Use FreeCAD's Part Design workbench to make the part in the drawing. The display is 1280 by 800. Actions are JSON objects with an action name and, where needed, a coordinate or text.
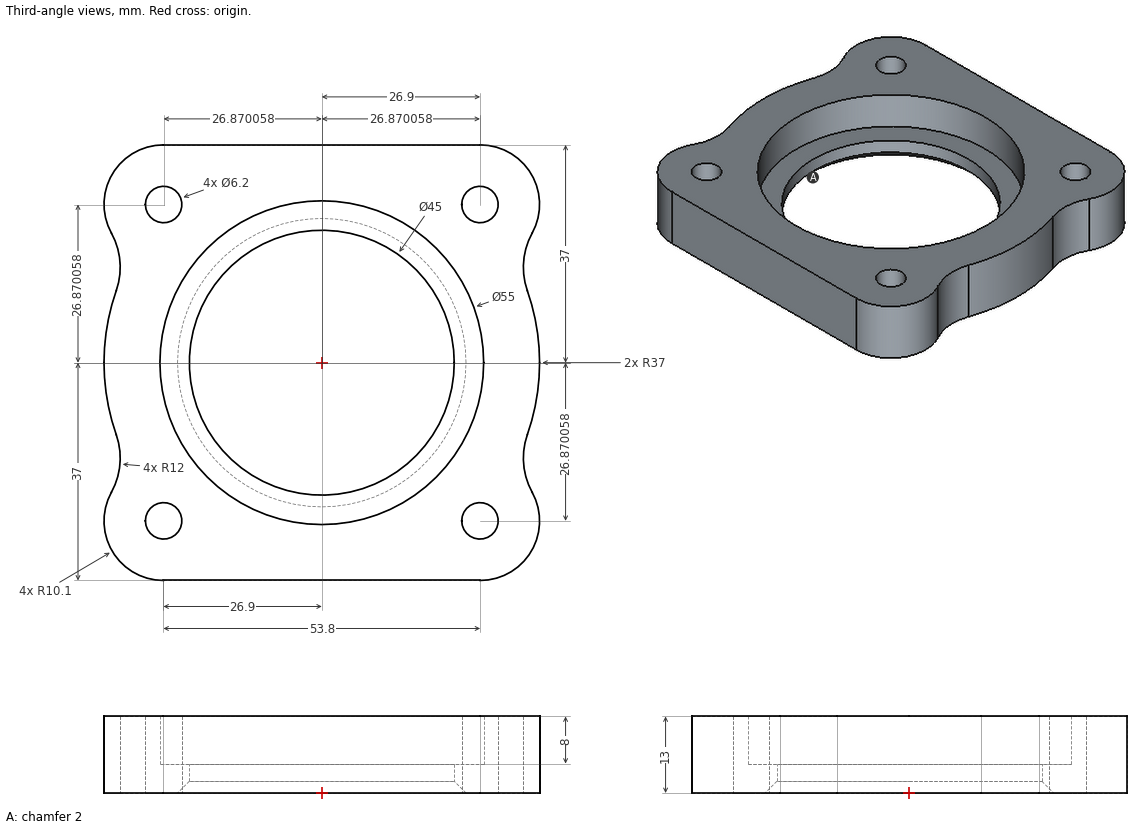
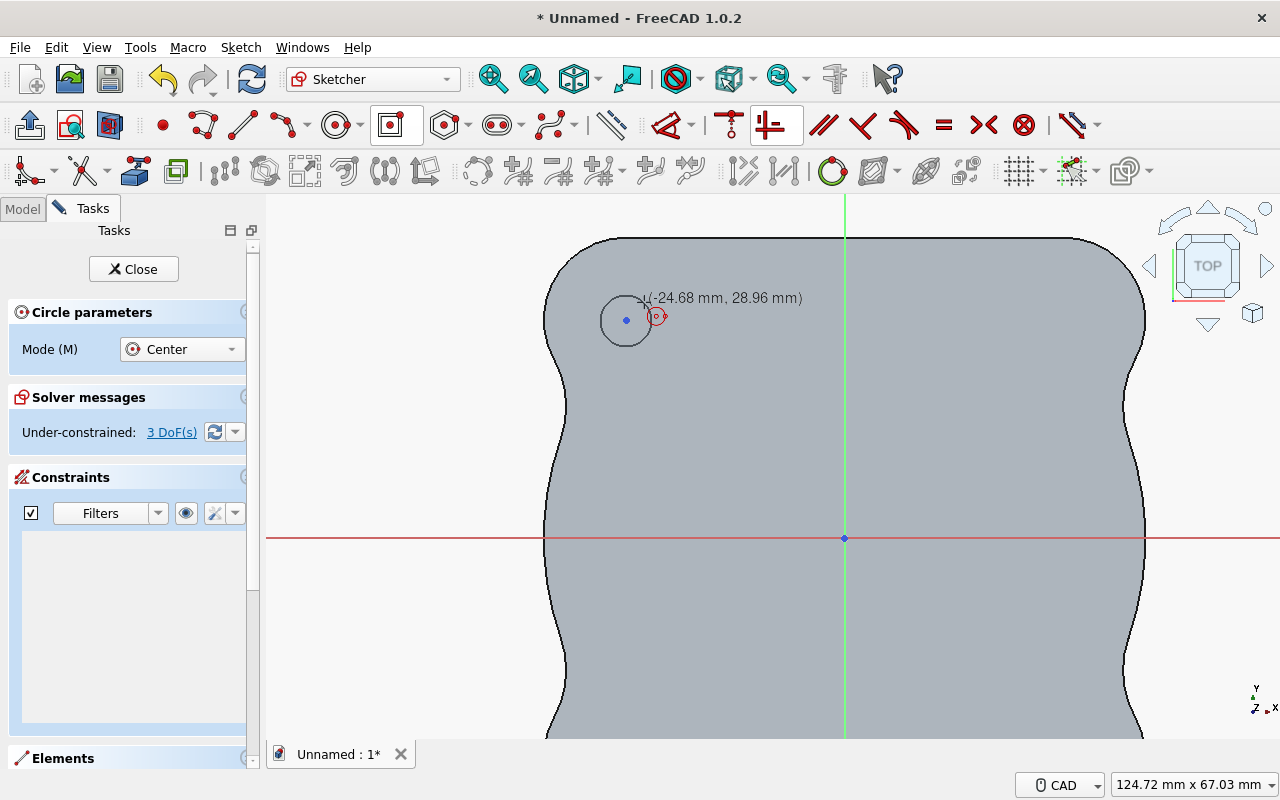
{"action": "left_click", "coordinate": [1063, 320]}
{"action": "left_click", "coordinate": [1081, 302]}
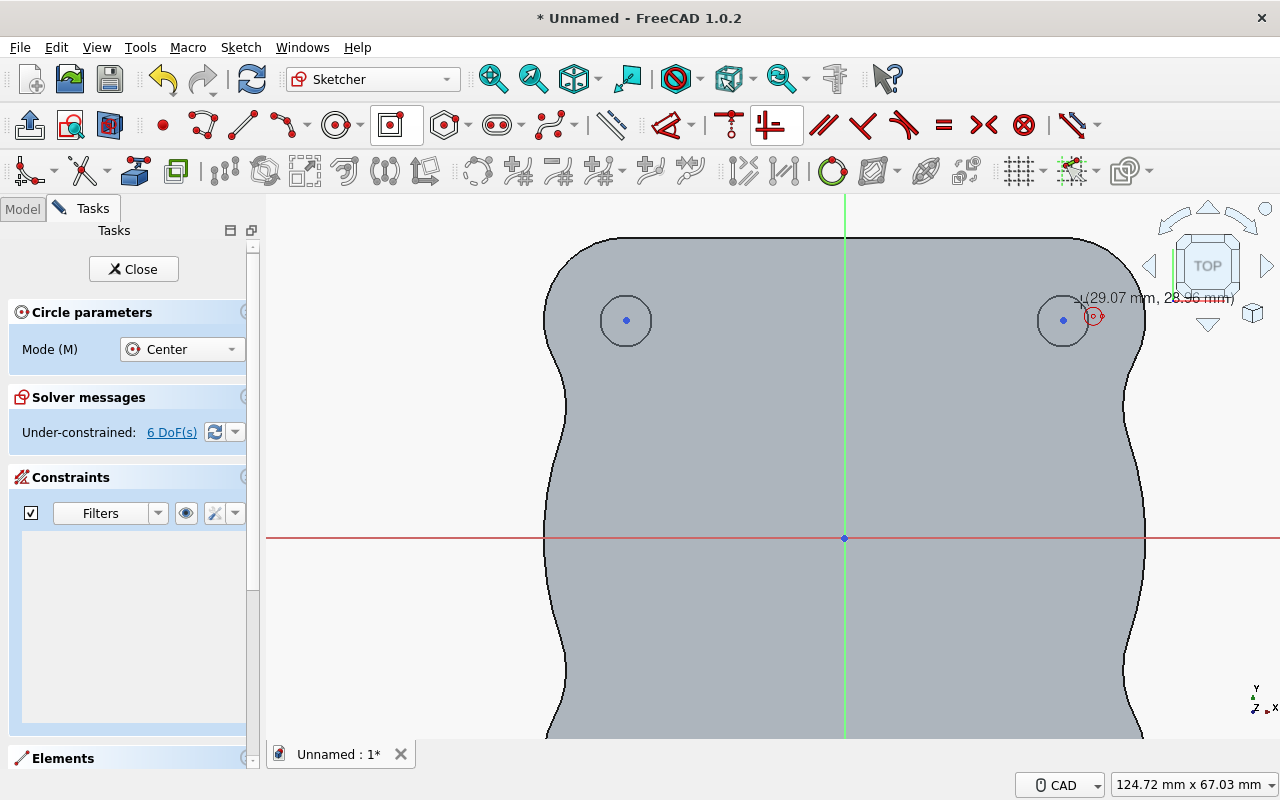
{"action": "scroll", "coordinate": [420, 320], "scroll_direction": "down", "scroll_amount": 2}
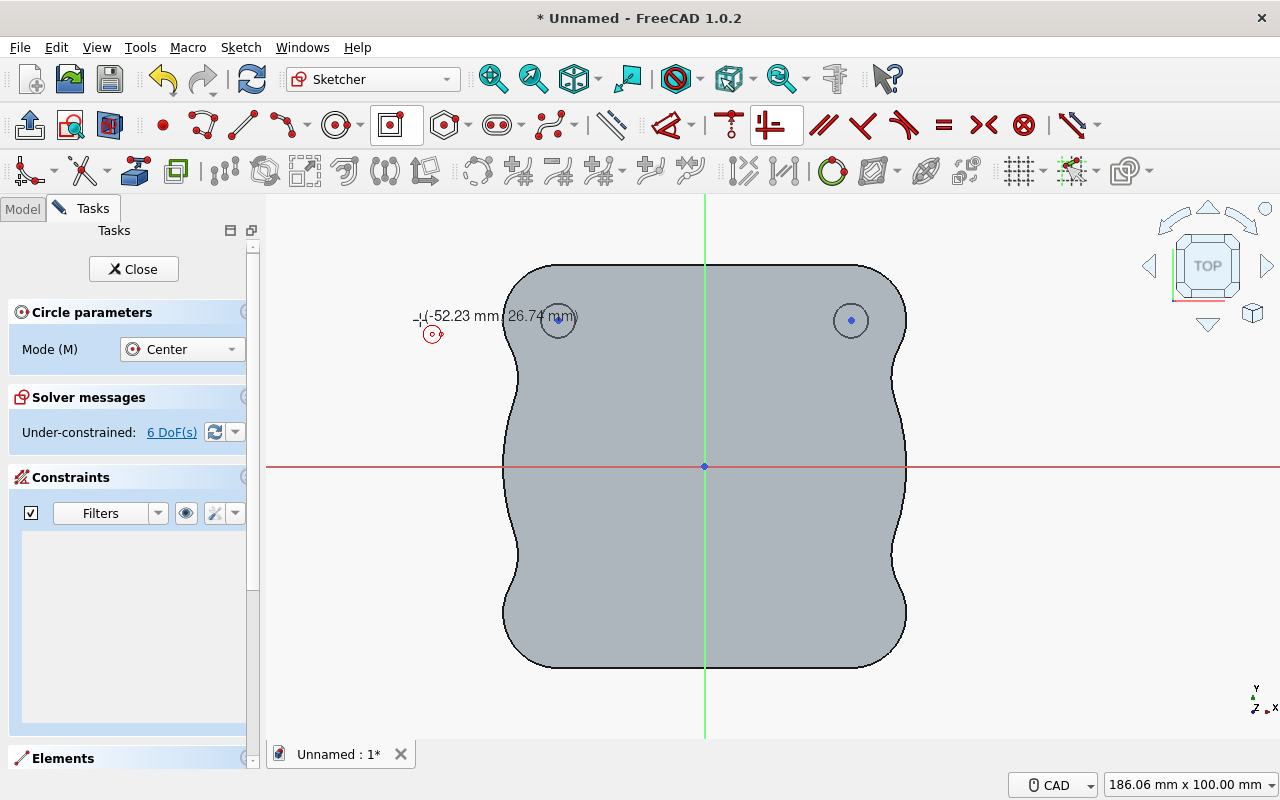
{"action": "scroll", "coordinate": [851, 613], "scroll_direction": "up", "scroll_amount": 2}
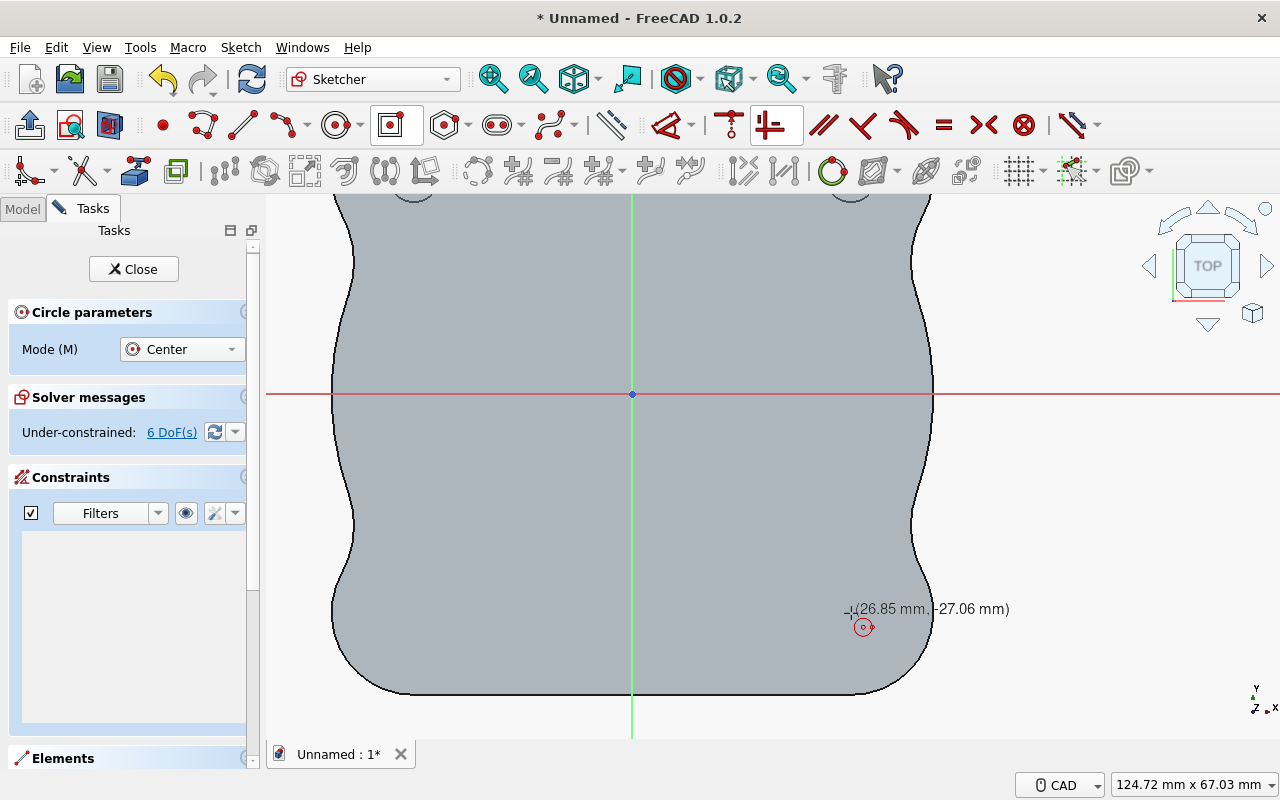
{"action": "left_click", "coordinate": [851, 613]}
{"action": "left_click", "coordinate": [869, 595]}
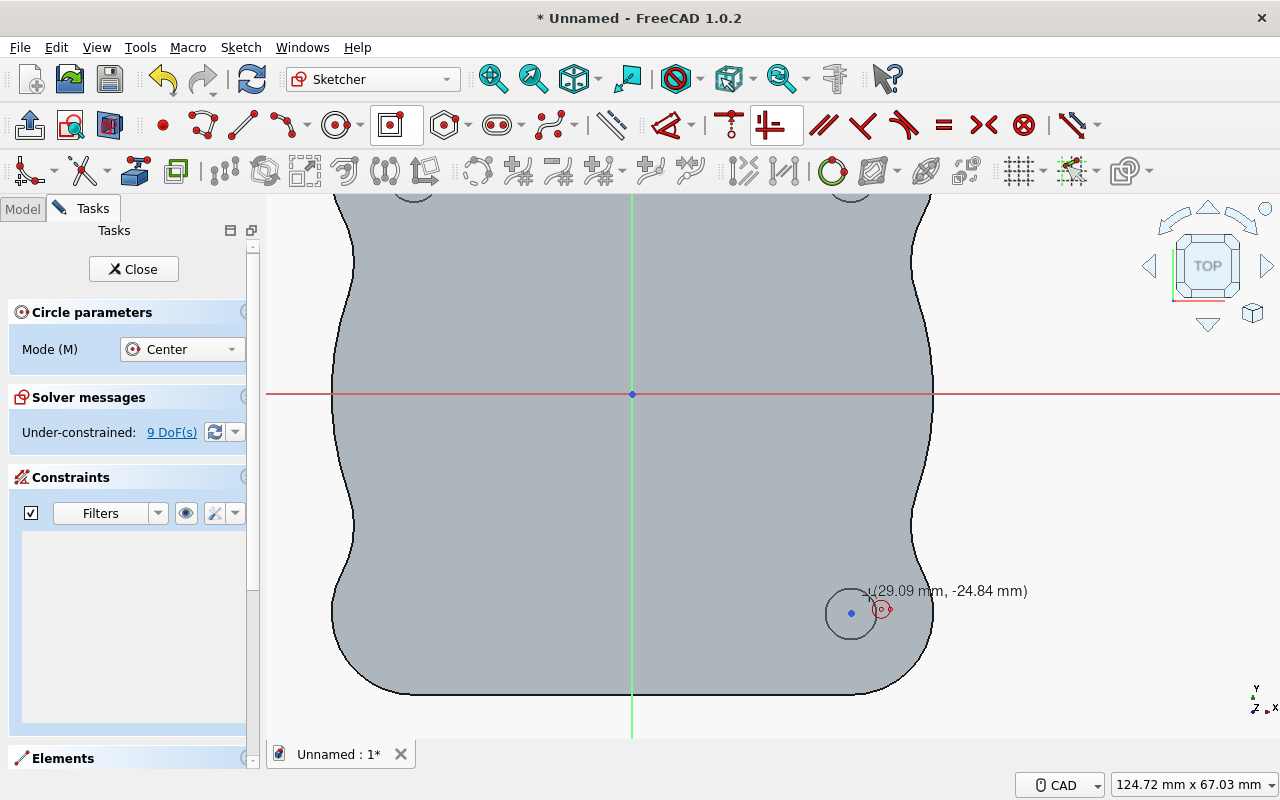
{"action": "left_click", "coordinate": [414, 613]}
{"action": "left_click", "coordinate": [432, 595]}
{"action": "key", "text": "Escape"}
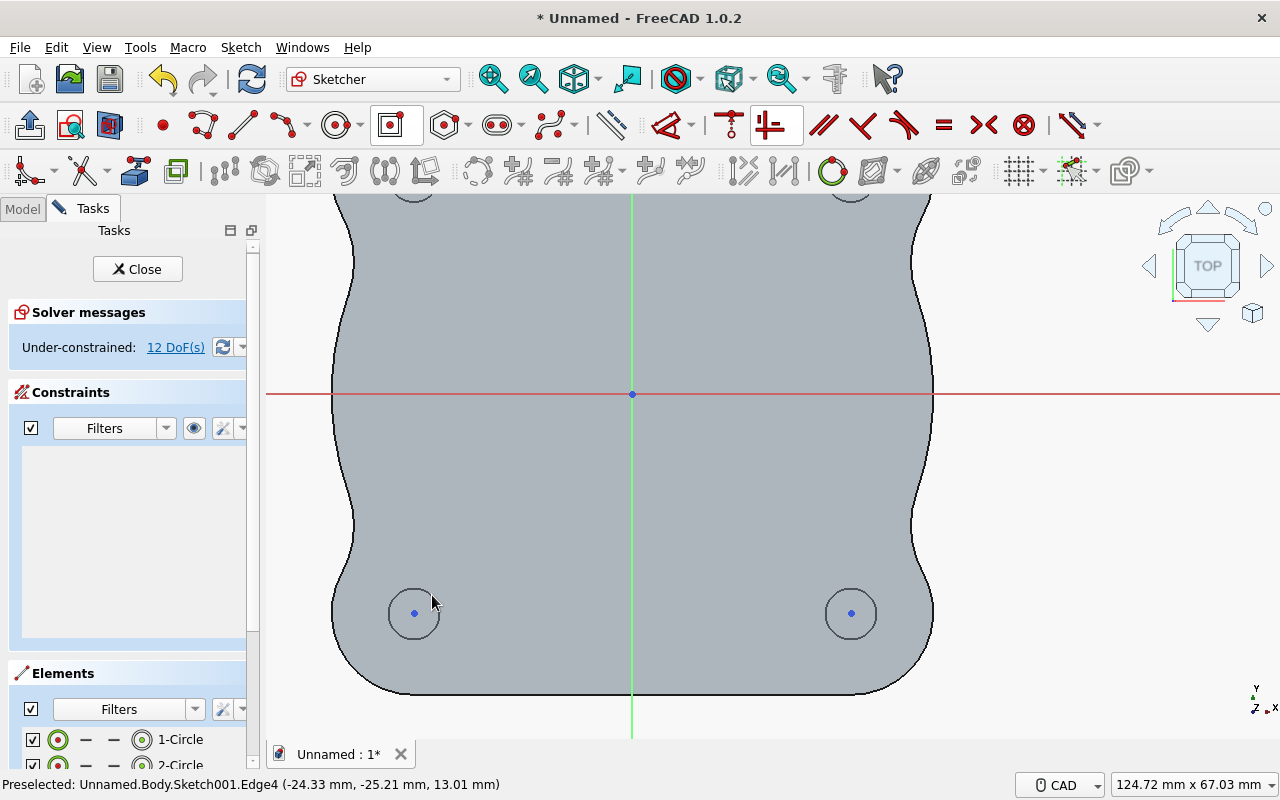
{"action": "scroll", "coordinate": [851, 614], "scroll_direction": "down", "scroll_amount": 2}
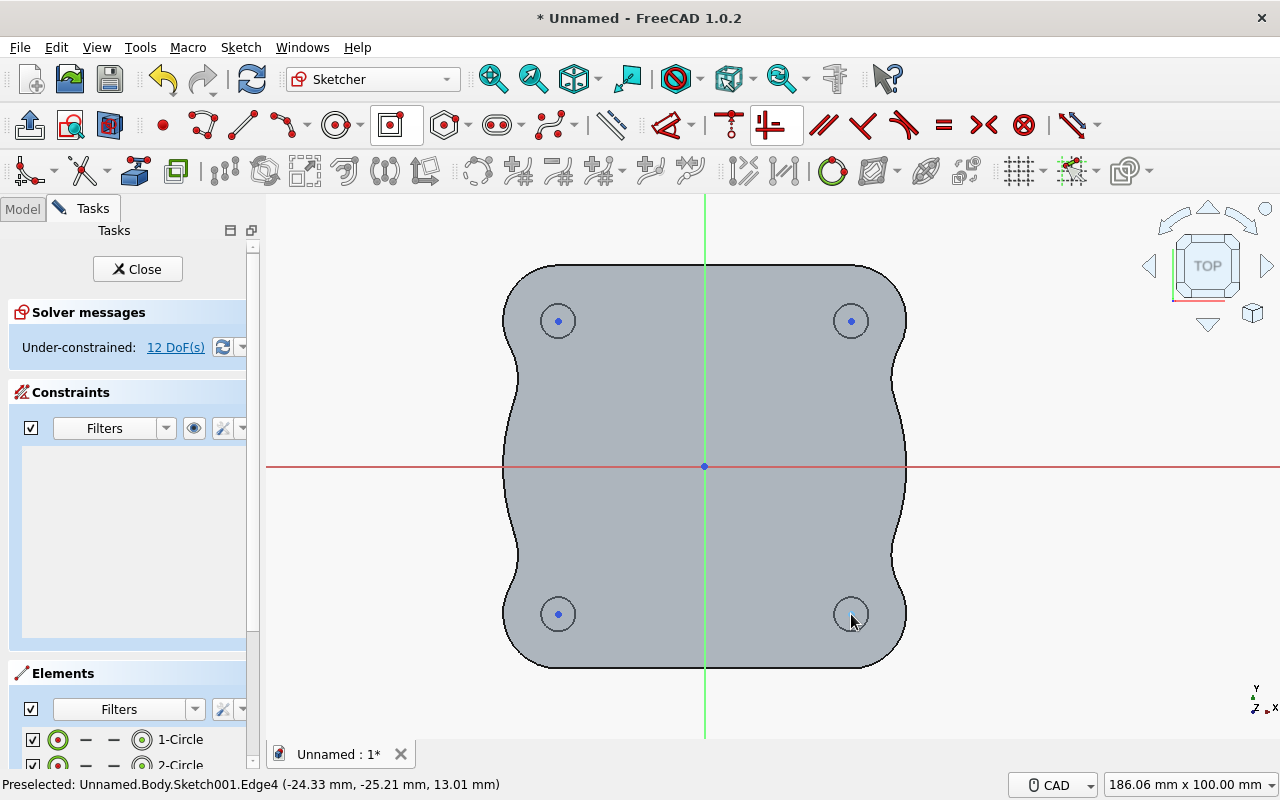
{"action": "left_click", "coordinate": [570, 309]}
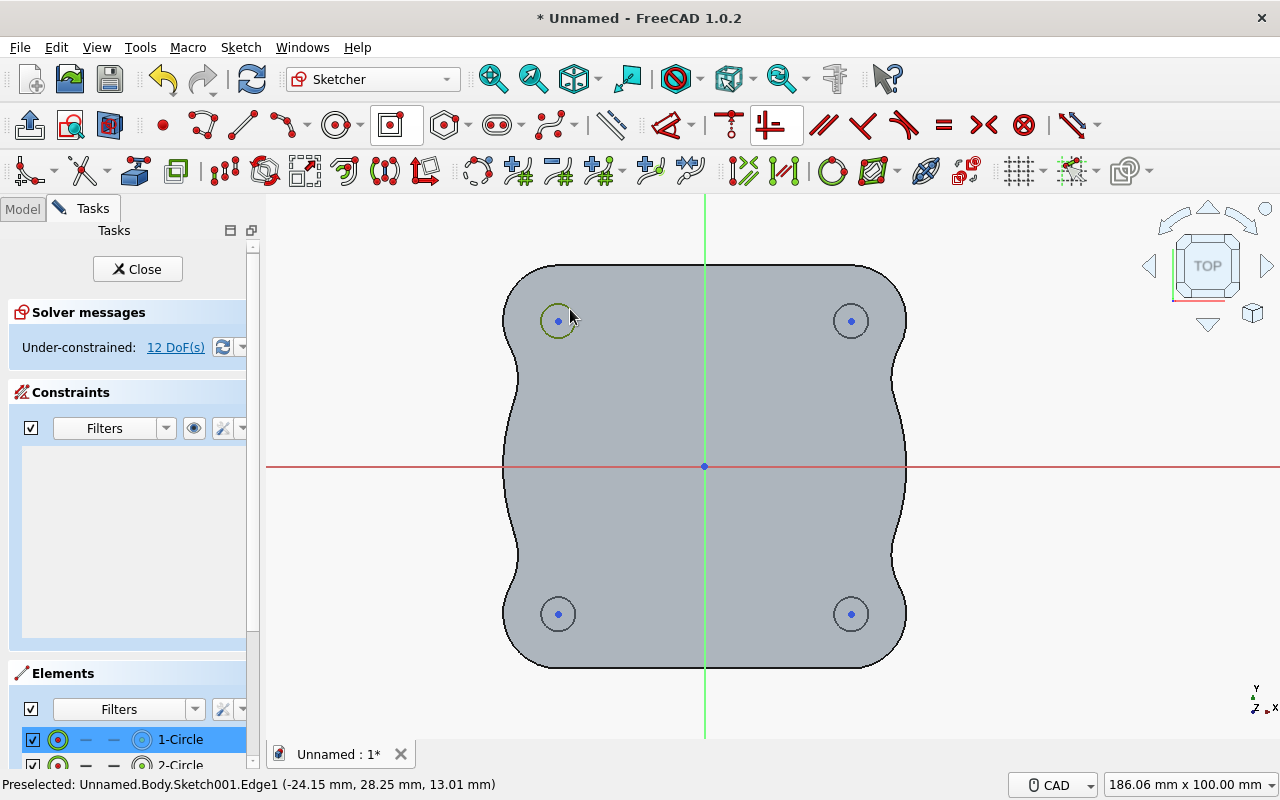
{"action": "left_click", "coordinate": [863, 309]}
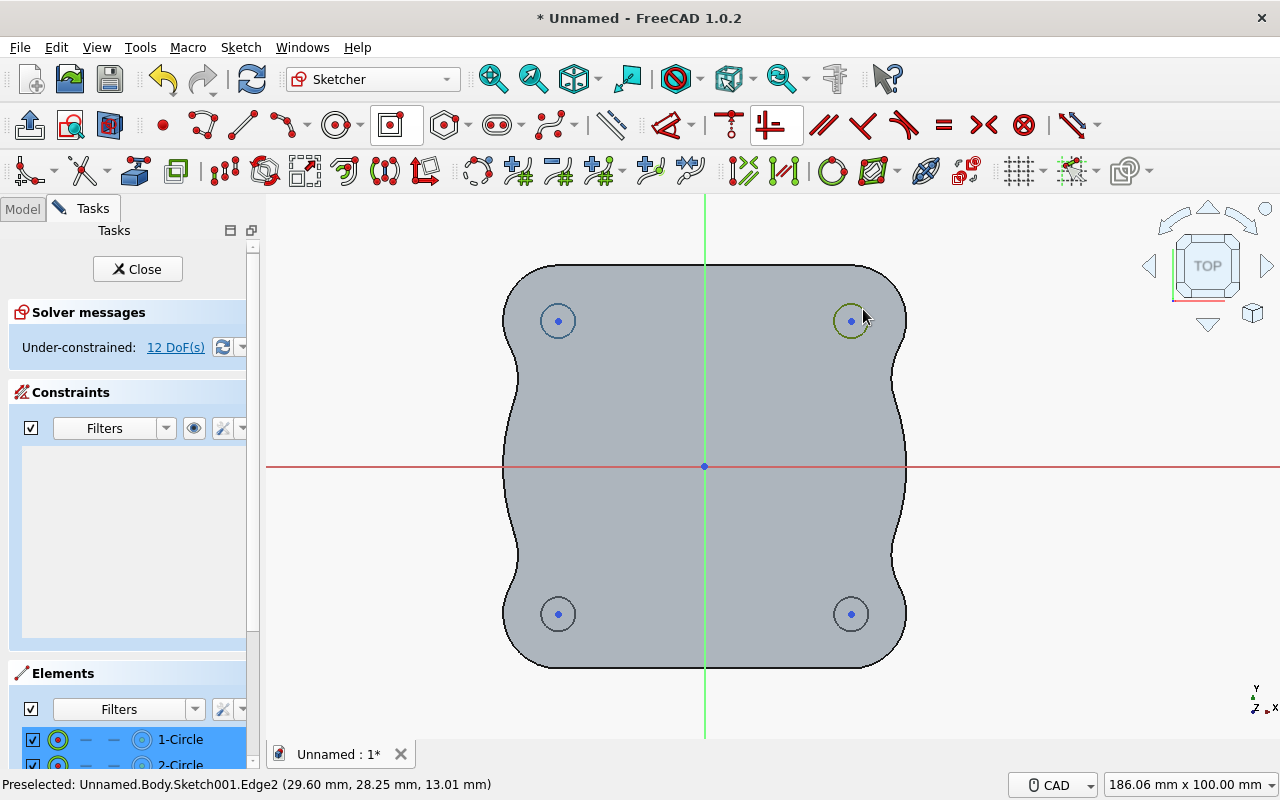
{"action": "left_click", "coordinate": [863, 602]}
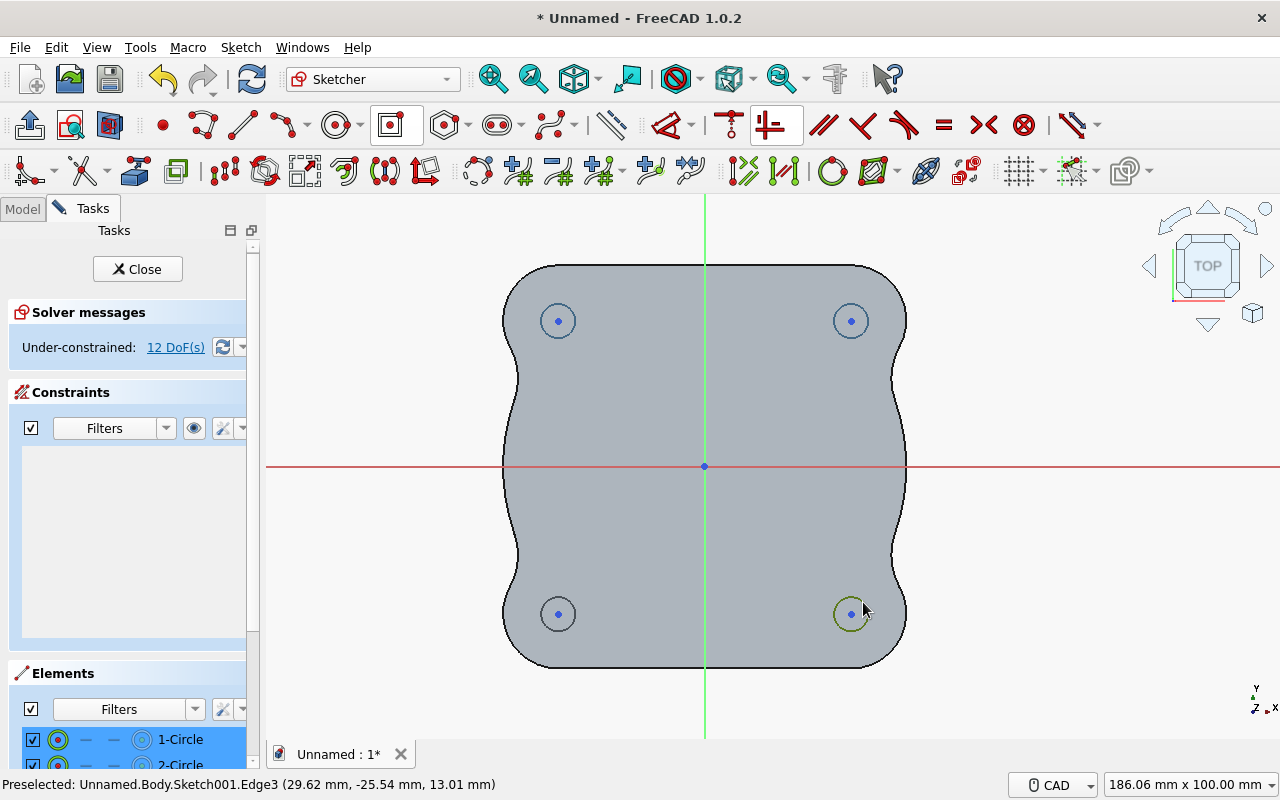
{"action": "left_click", "coordinate": [570, 602]}